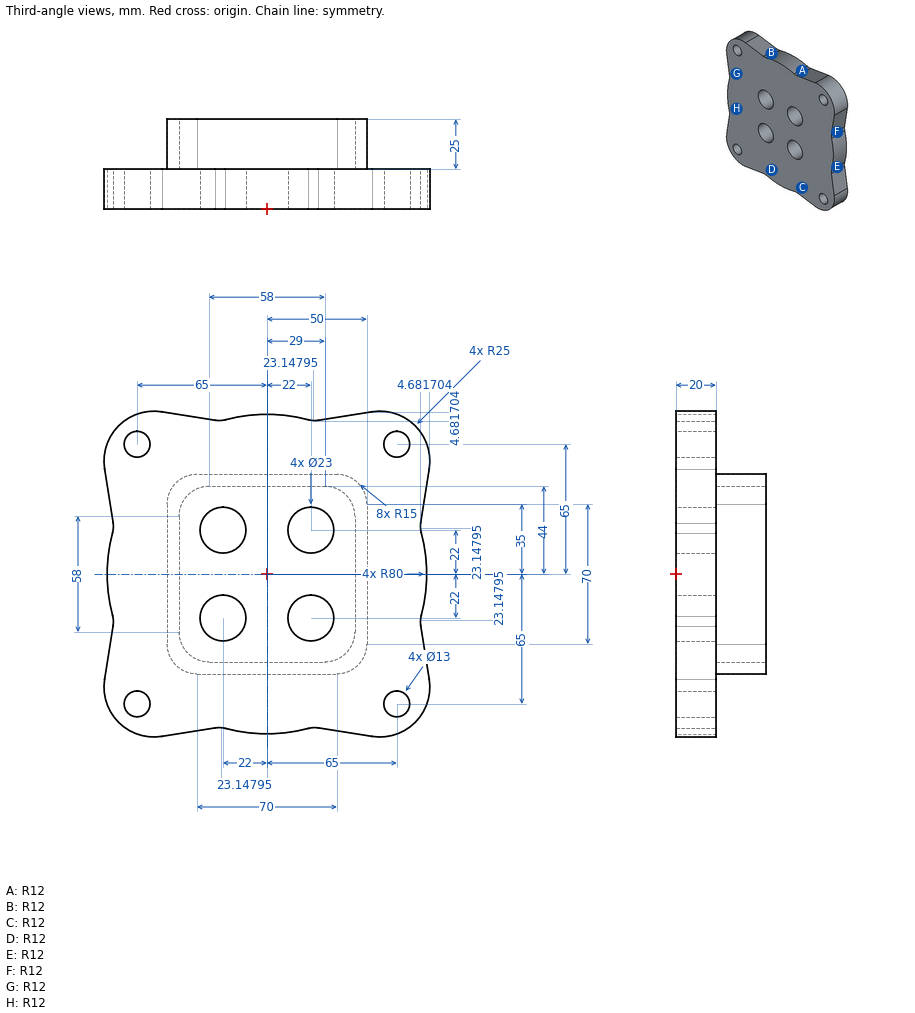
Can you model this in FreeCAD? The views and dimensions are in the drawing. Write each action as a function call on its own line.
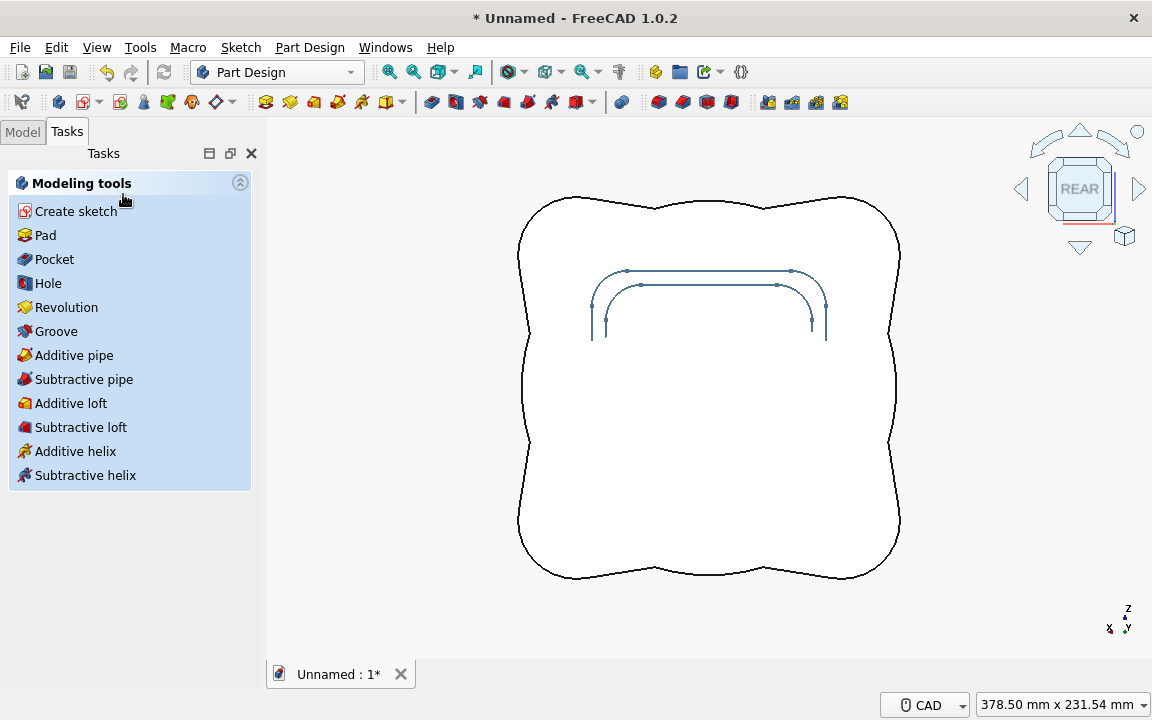
click(266, 102)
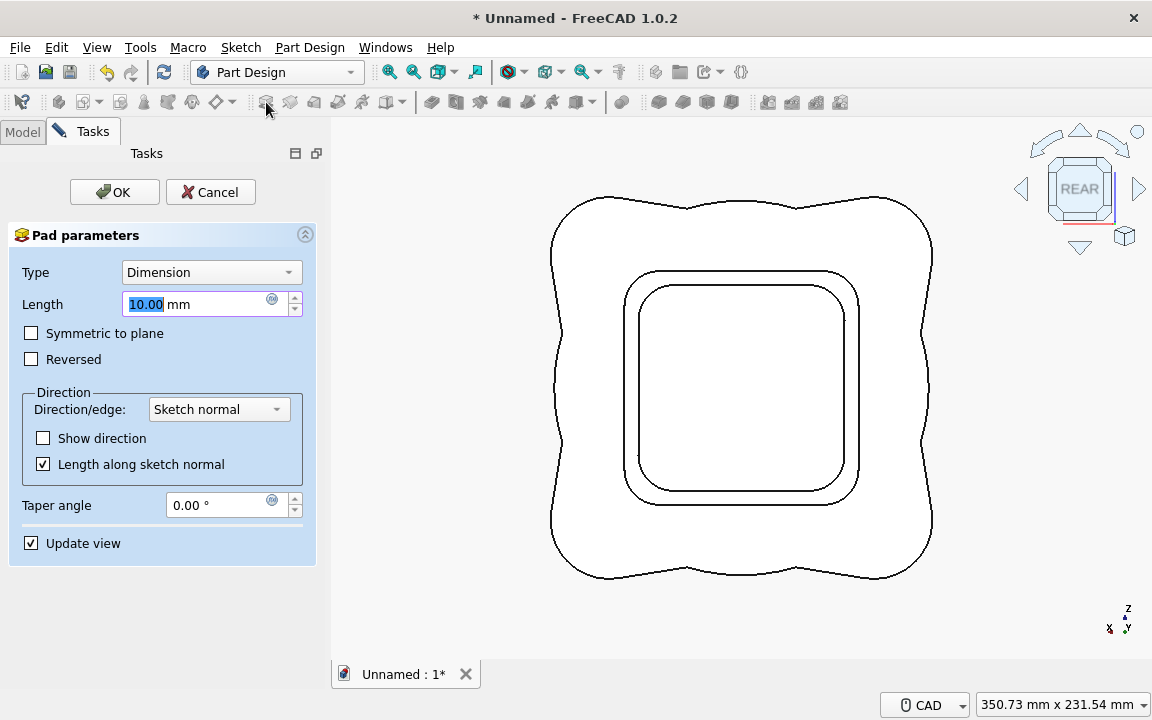
text(25)
key(Tab)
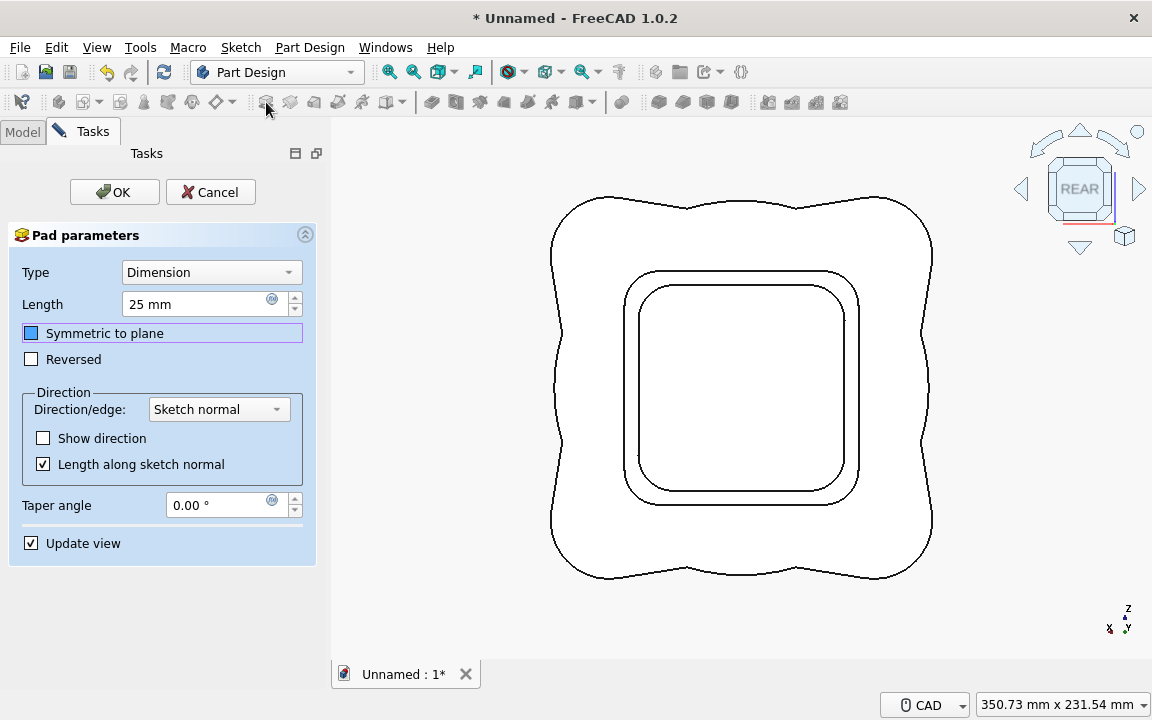
click(115, 192)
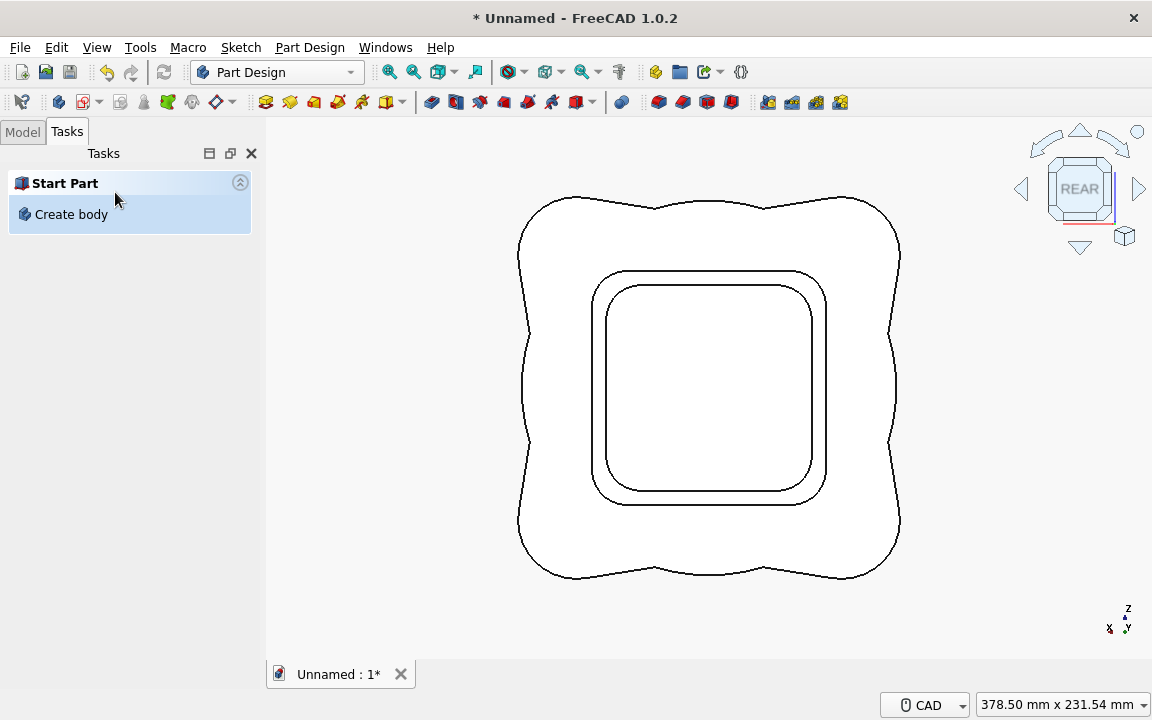
click(873, 496)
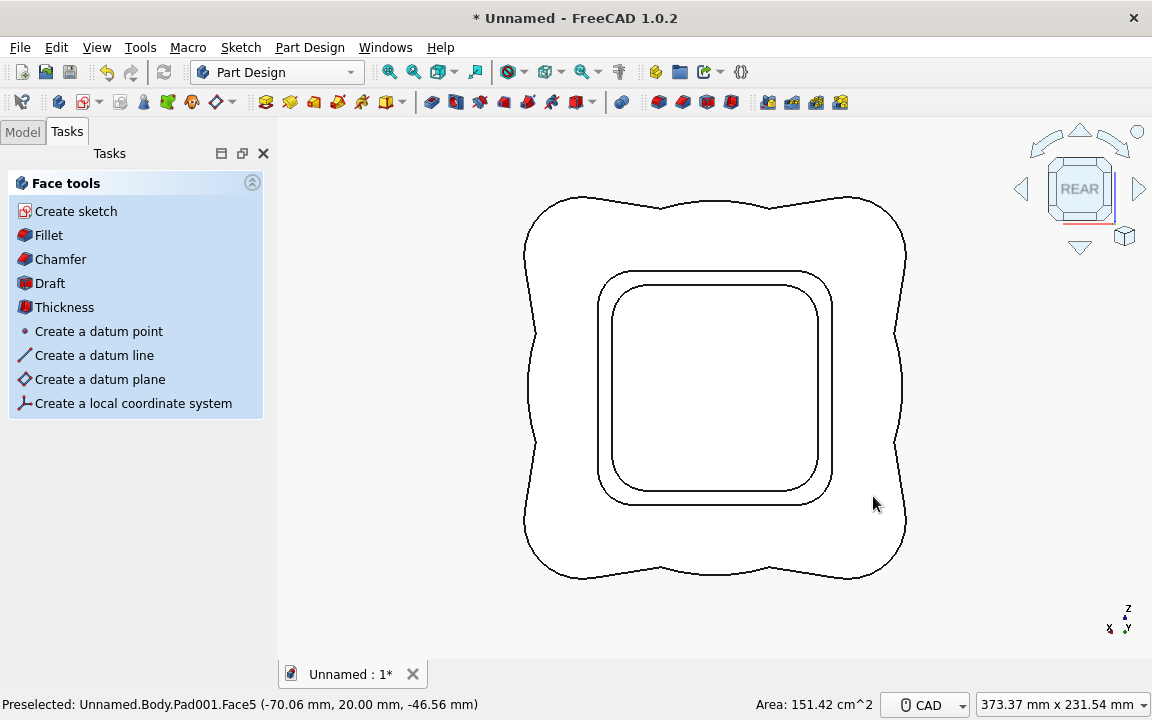
click(84, 102)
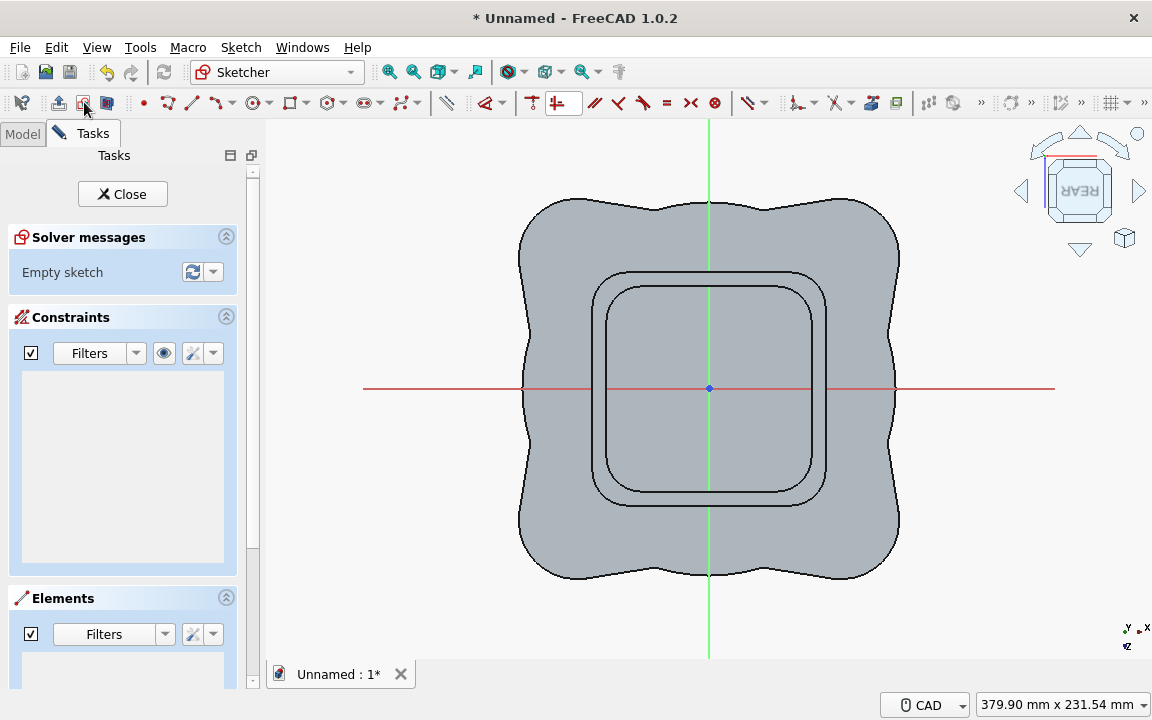
scroll(765, 389, up, 4)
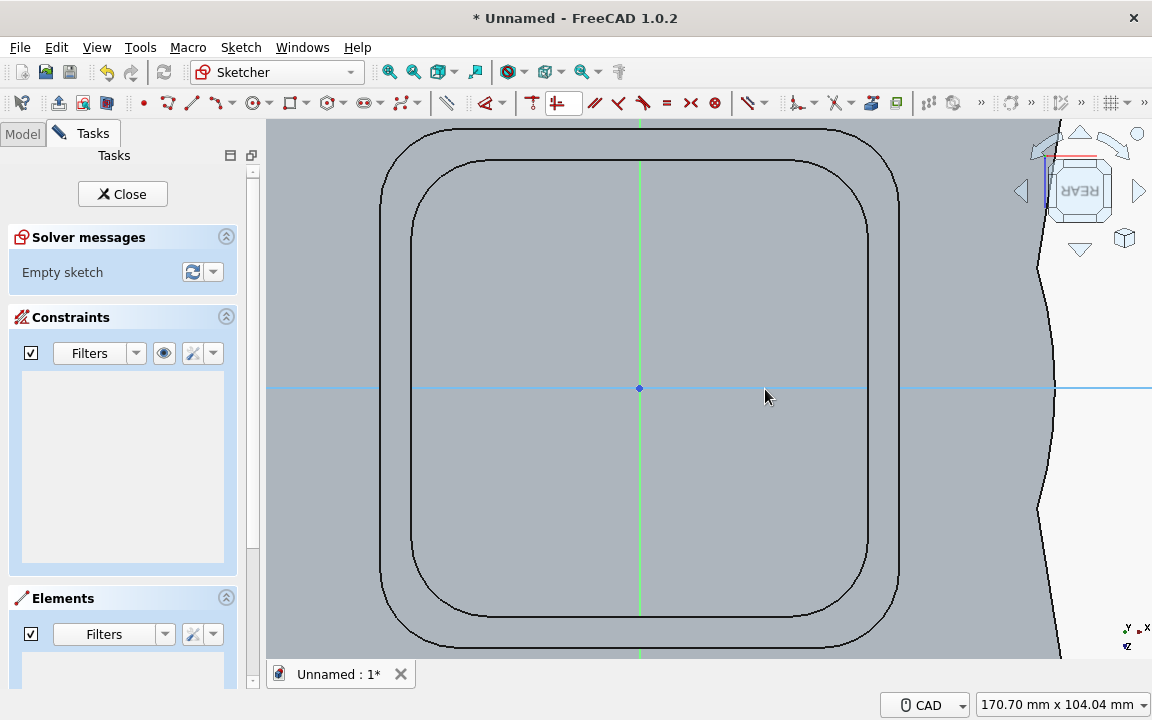
click(254, 104)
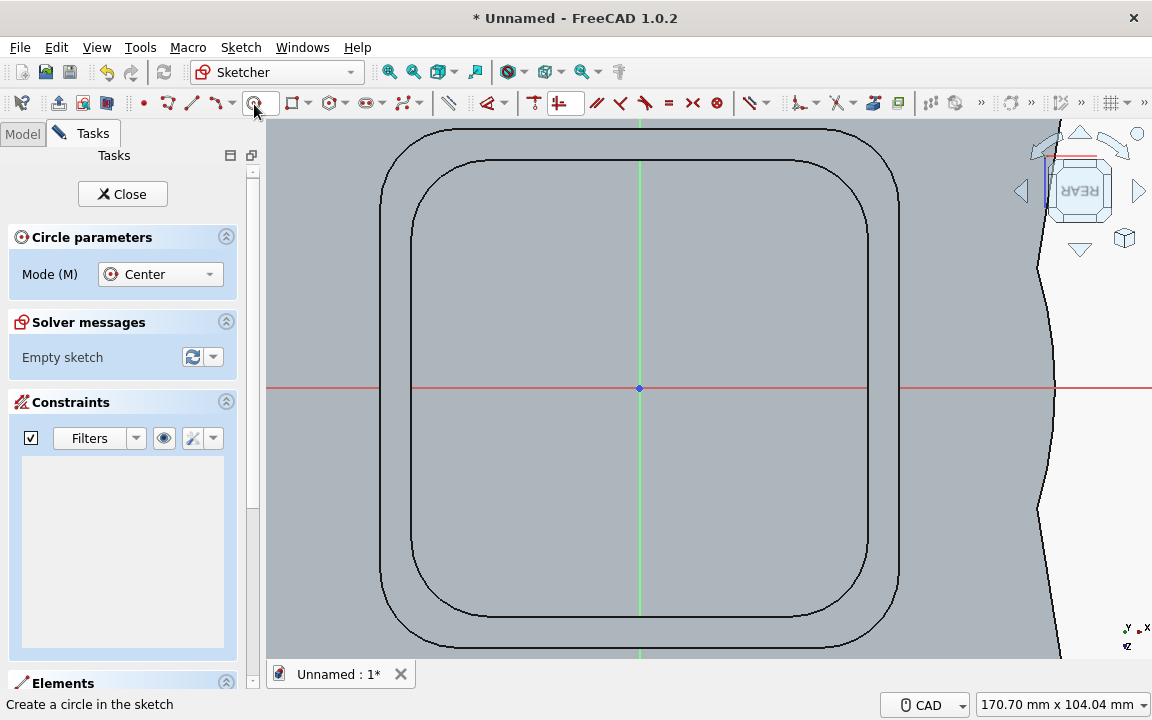
click(754, 503)
move(796, 460)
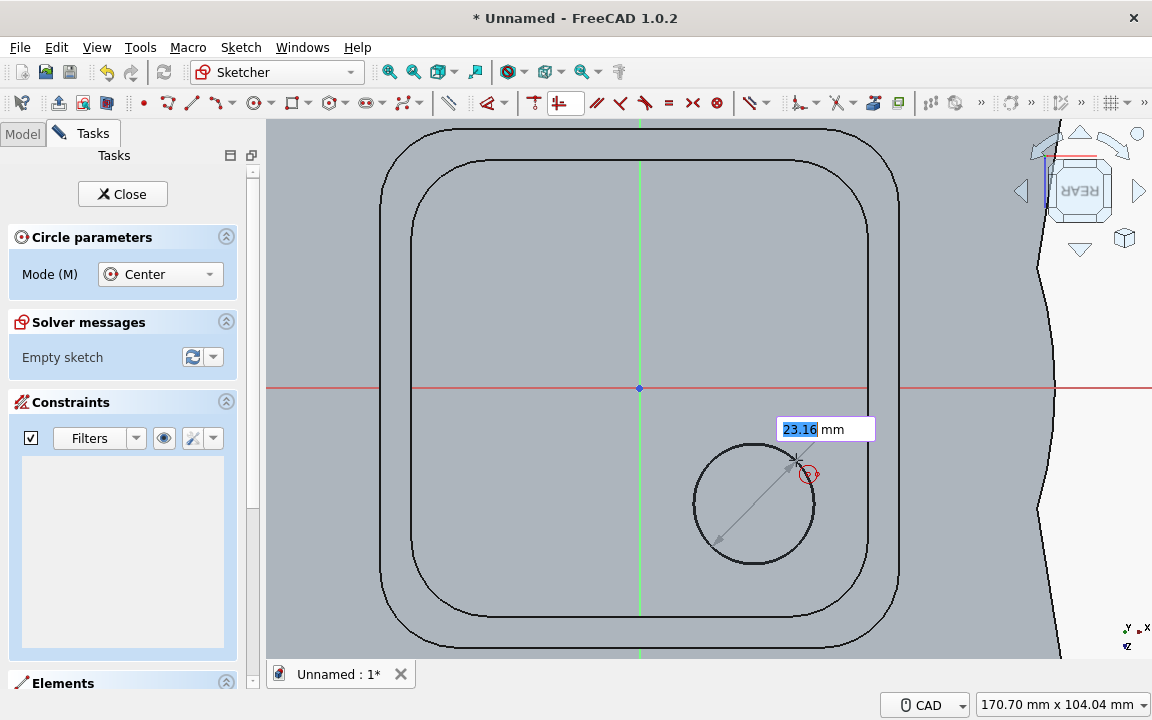
text(23)
key(Return)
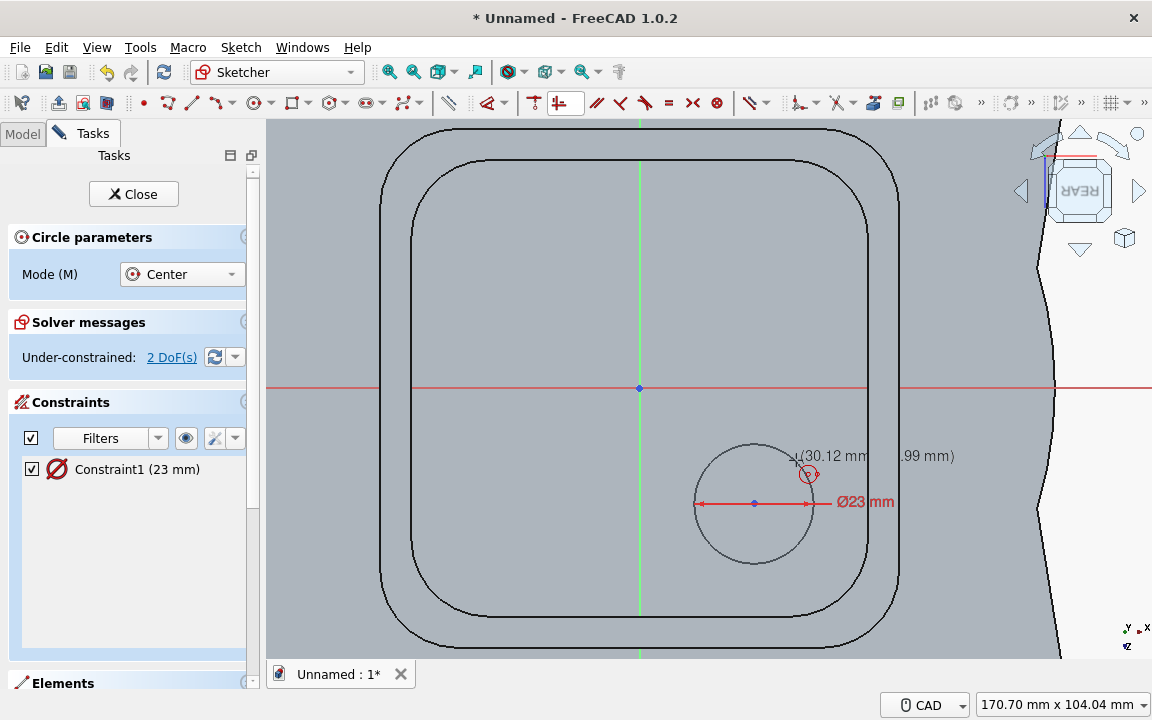
click(754, 274)
move(796, 232)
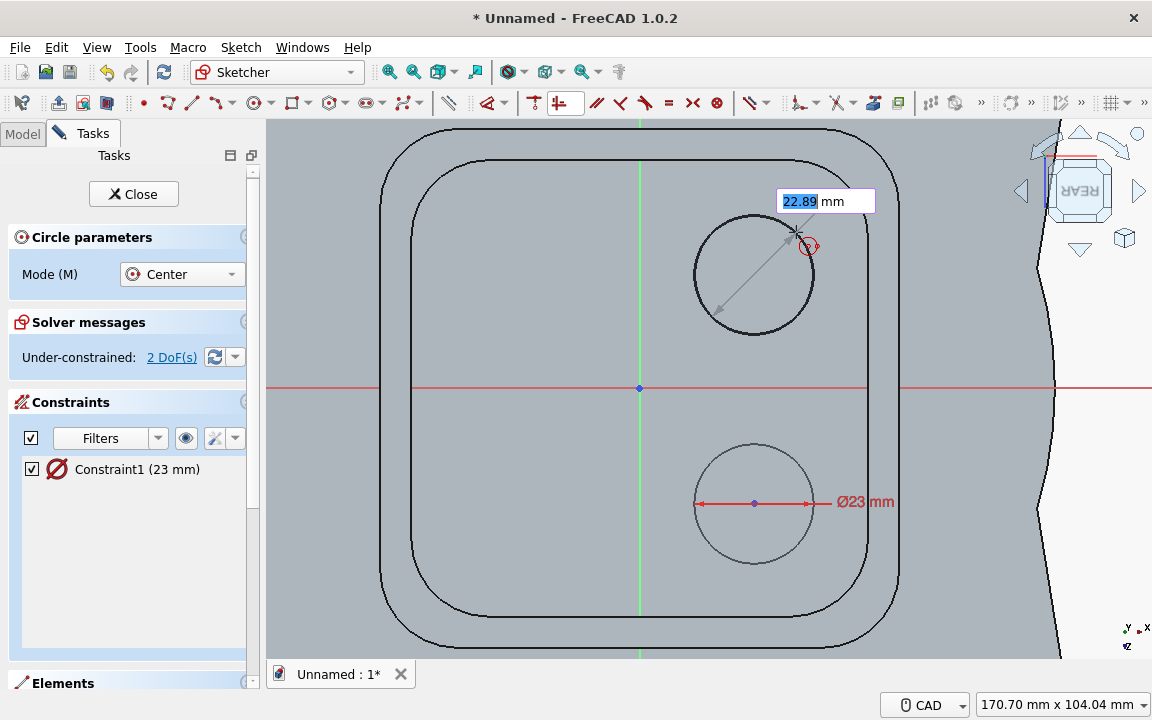
text(23)
key(Return)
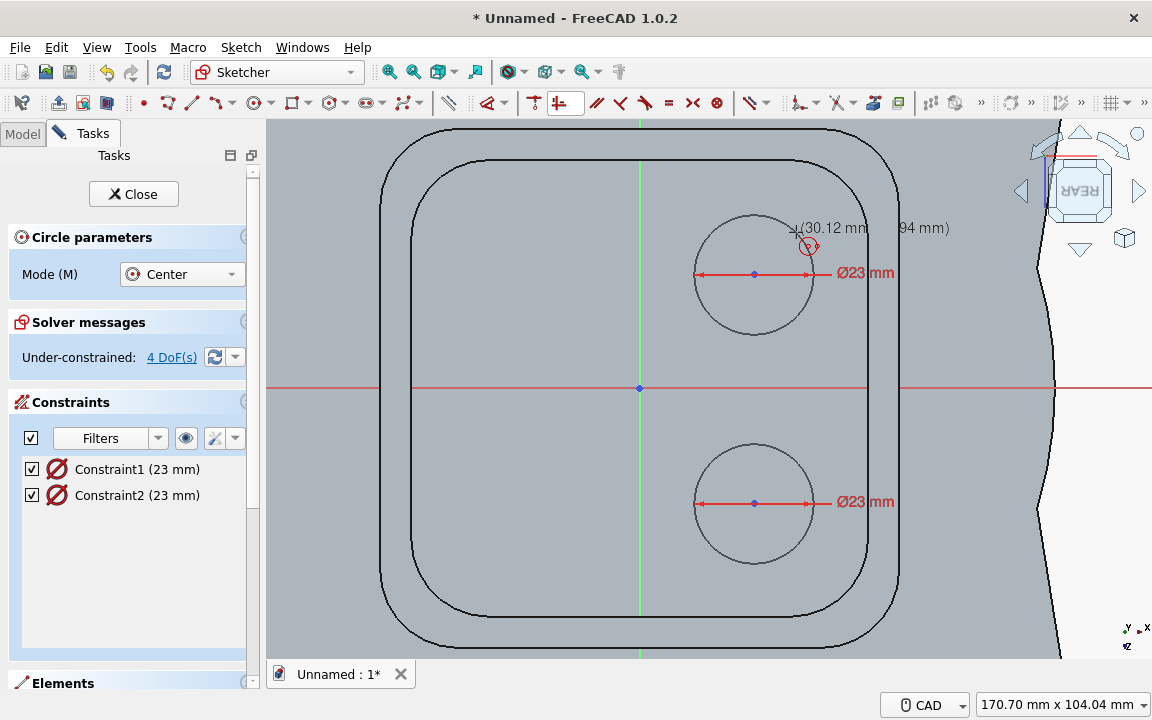
click(525, 274)
move(568, 232)